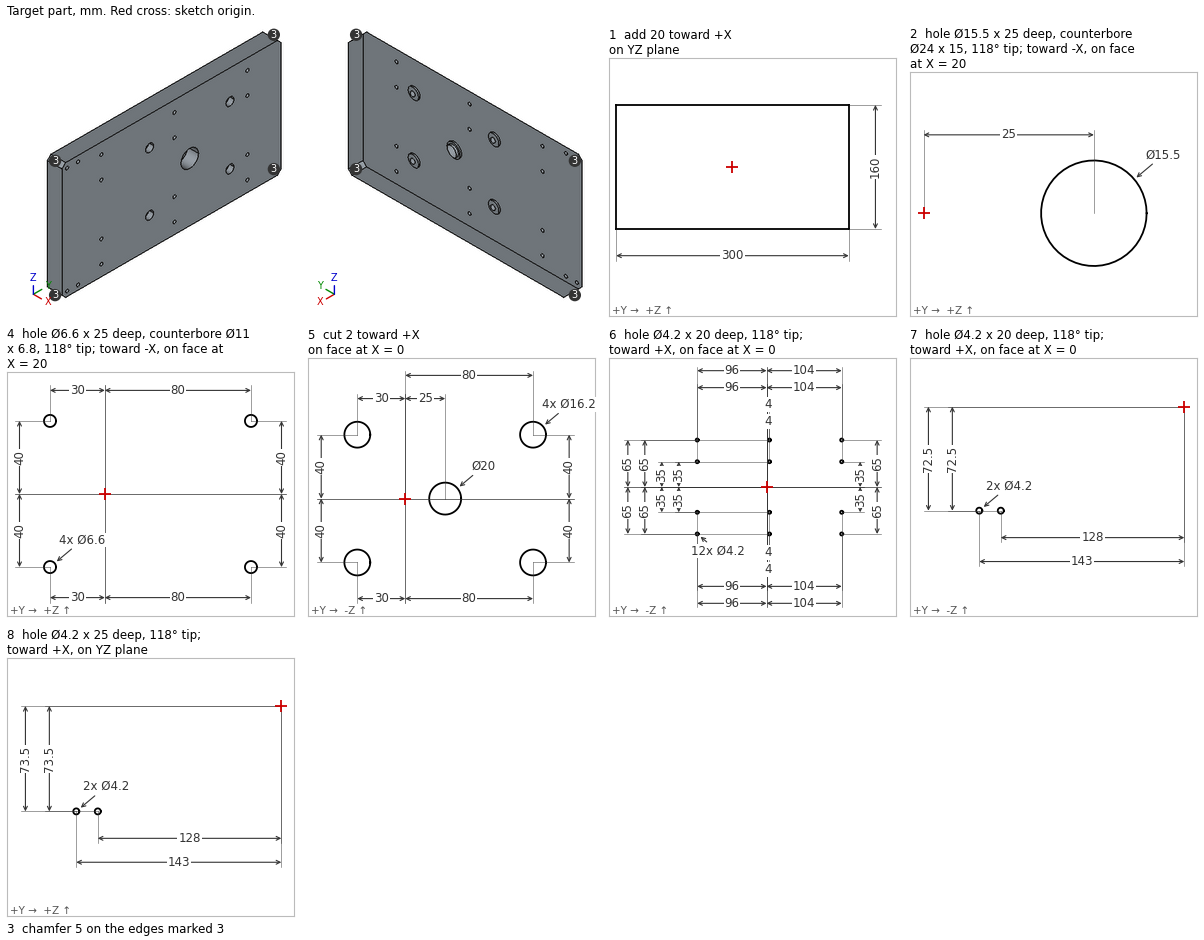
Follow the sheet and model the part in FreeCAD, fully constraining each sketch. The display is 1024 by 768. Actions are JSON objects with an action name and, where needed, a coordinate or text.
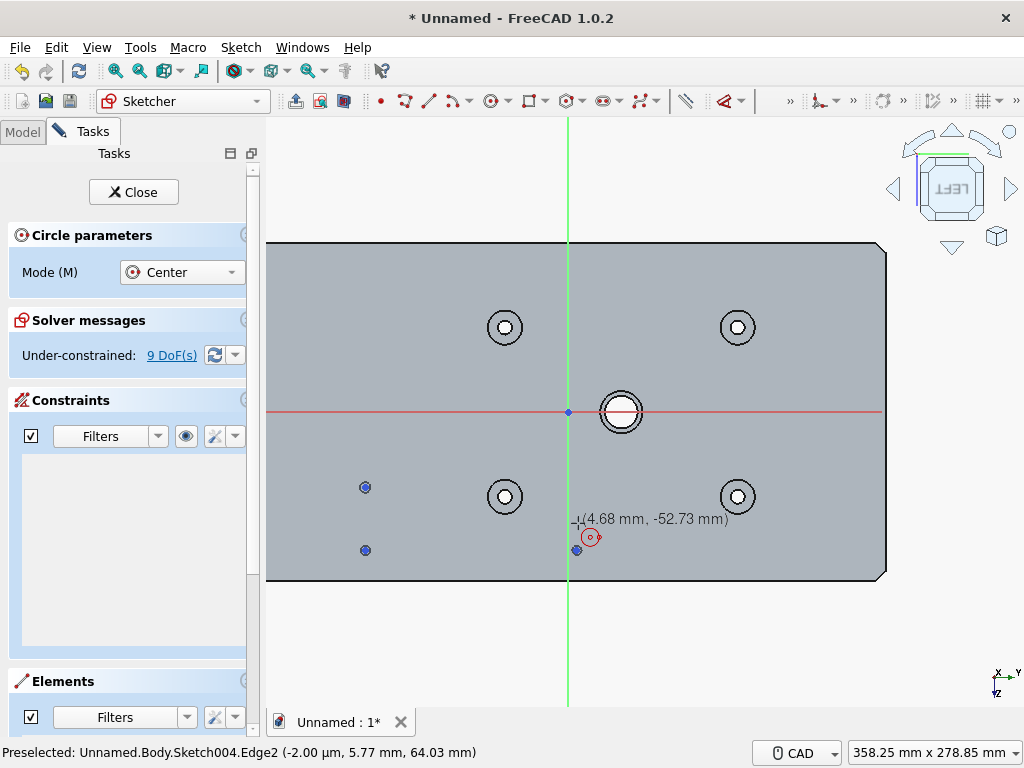
{"action": "scroll", "coordinate": [577, 486], "scroll_direction": "up", "scroll_amount": 4}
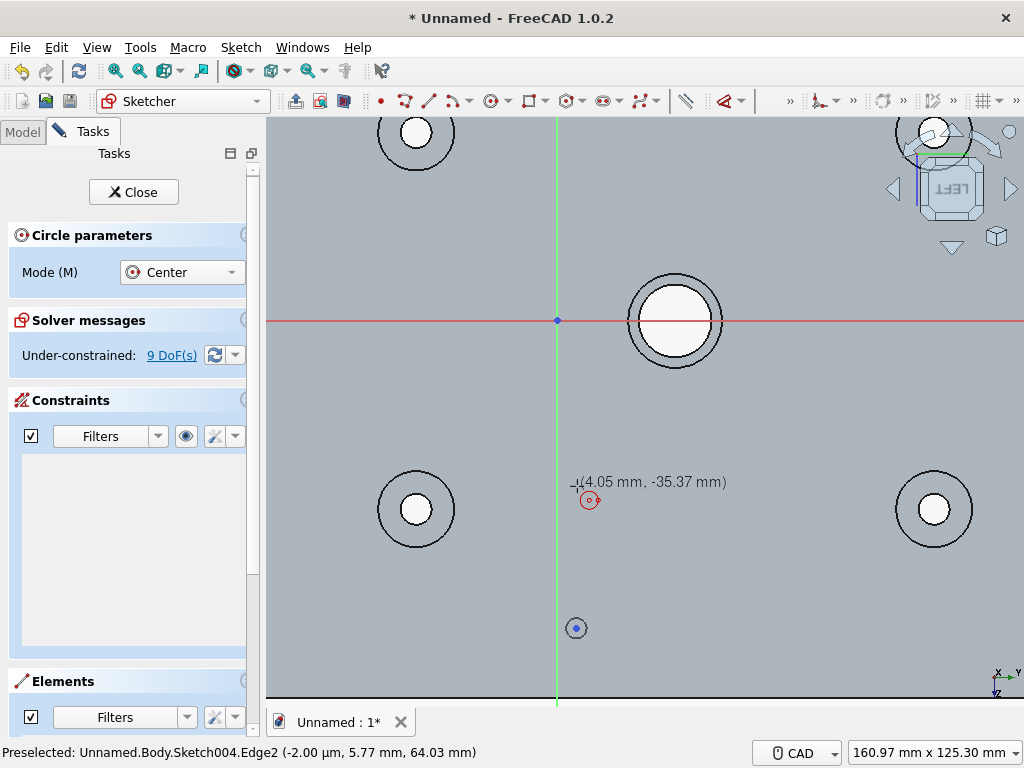
{"action": "left_click", "coordinate": [576, 486]}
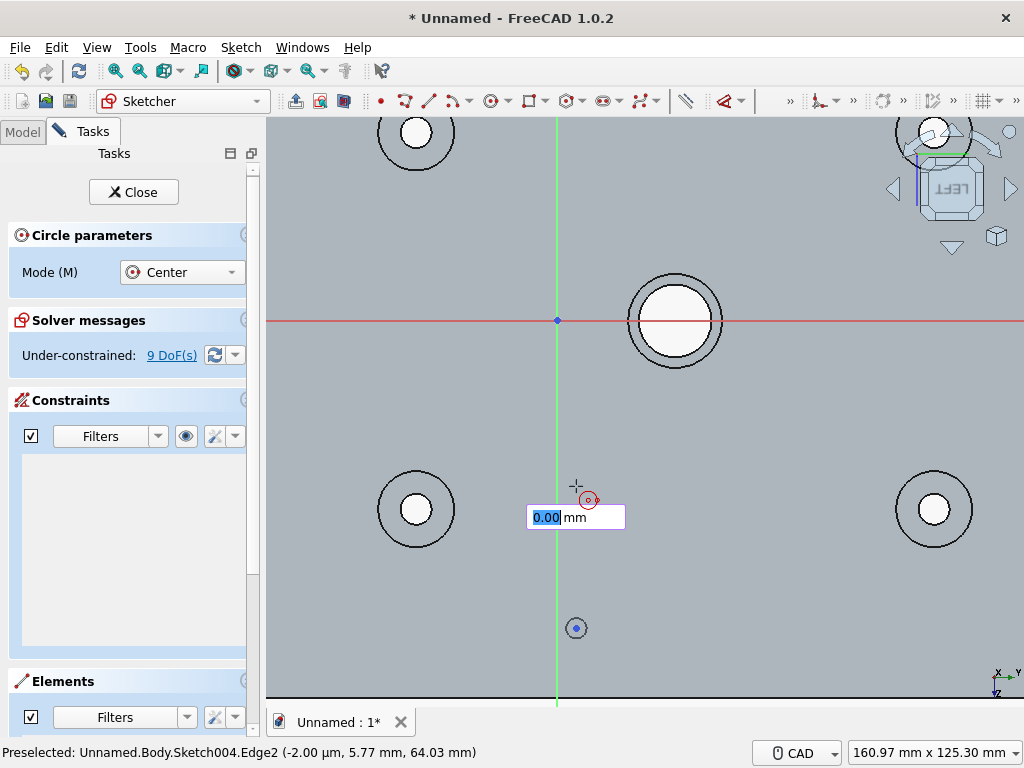
{"action": "scroll", "coordinate": [583, 479], "scroll_direction": "up", "scroll_amount": 3}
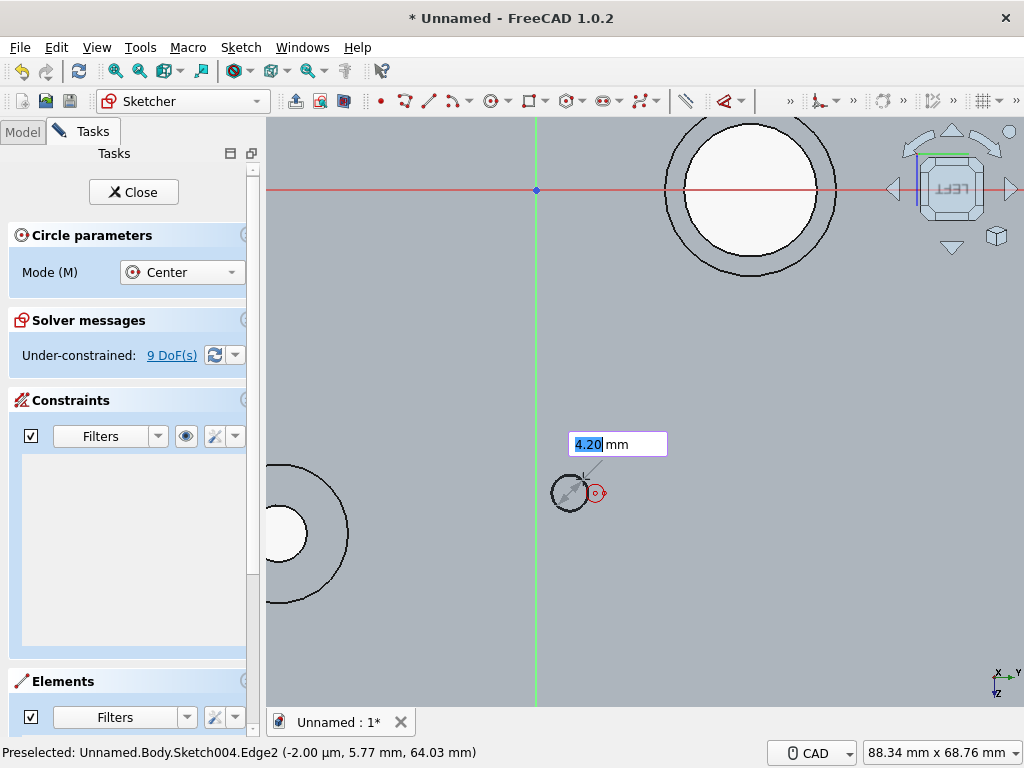
{"action": "left_click", "coordinate": [583, 478]}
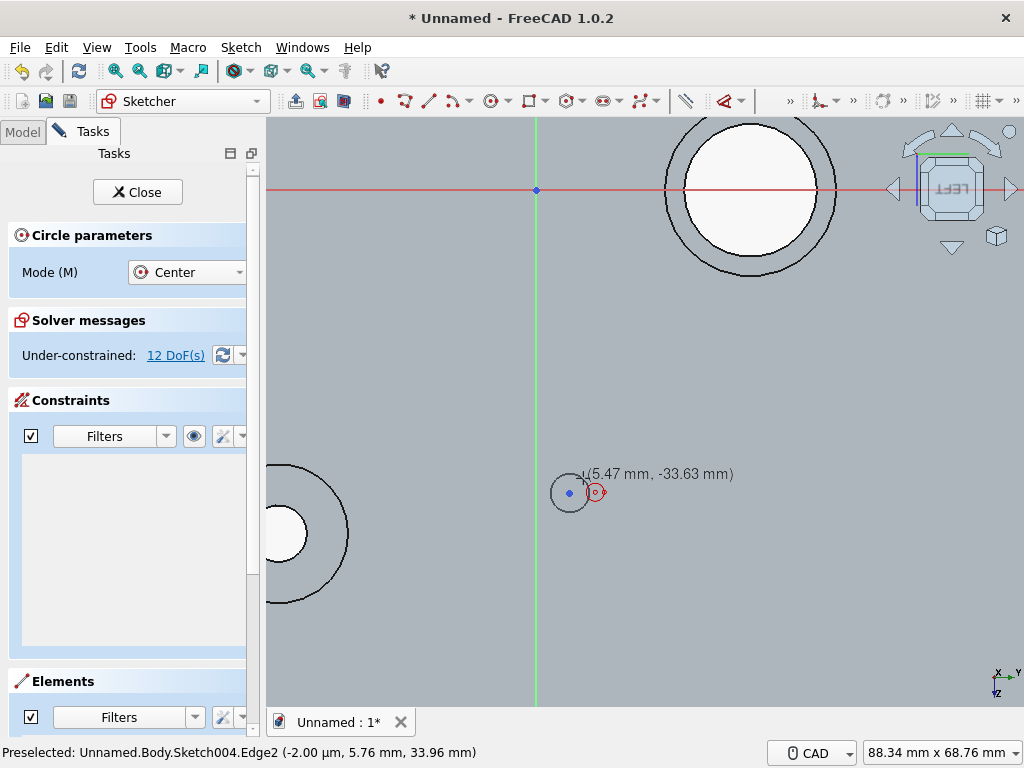
{"action": "scroll", "coordinate": [579, 485], "scroll_direction": "down", "scroll_amount": 7}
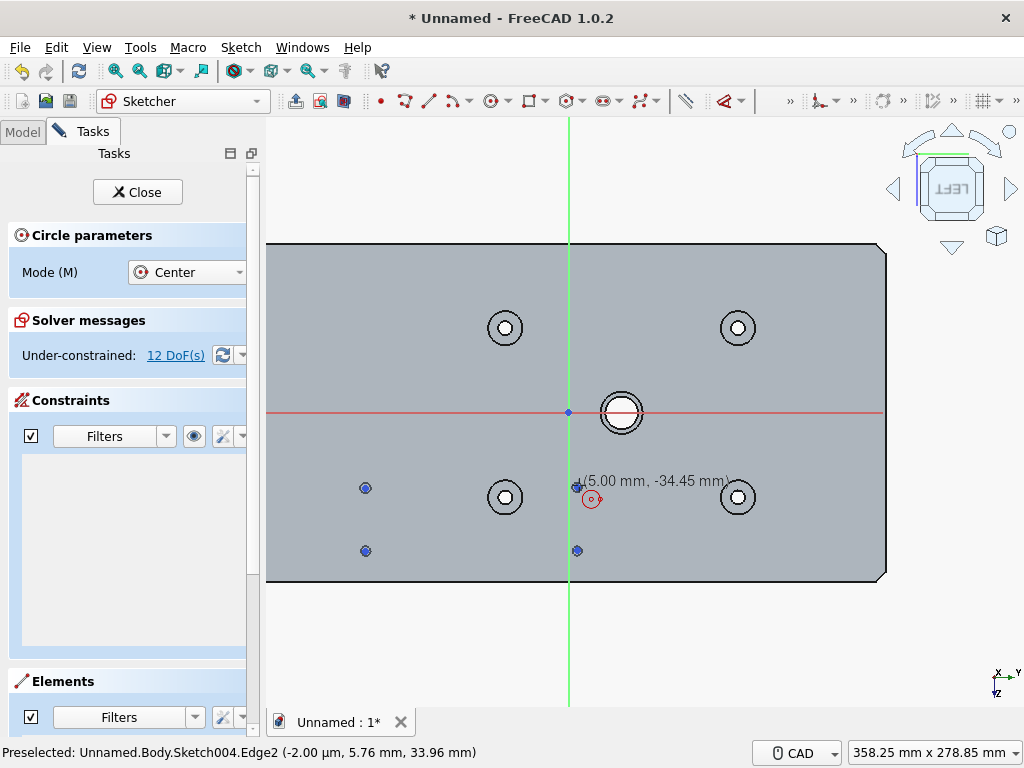
{"action": "scroll", "coordinate": [789, 550], "scroll_direction": "up", "scroll_amount": 9}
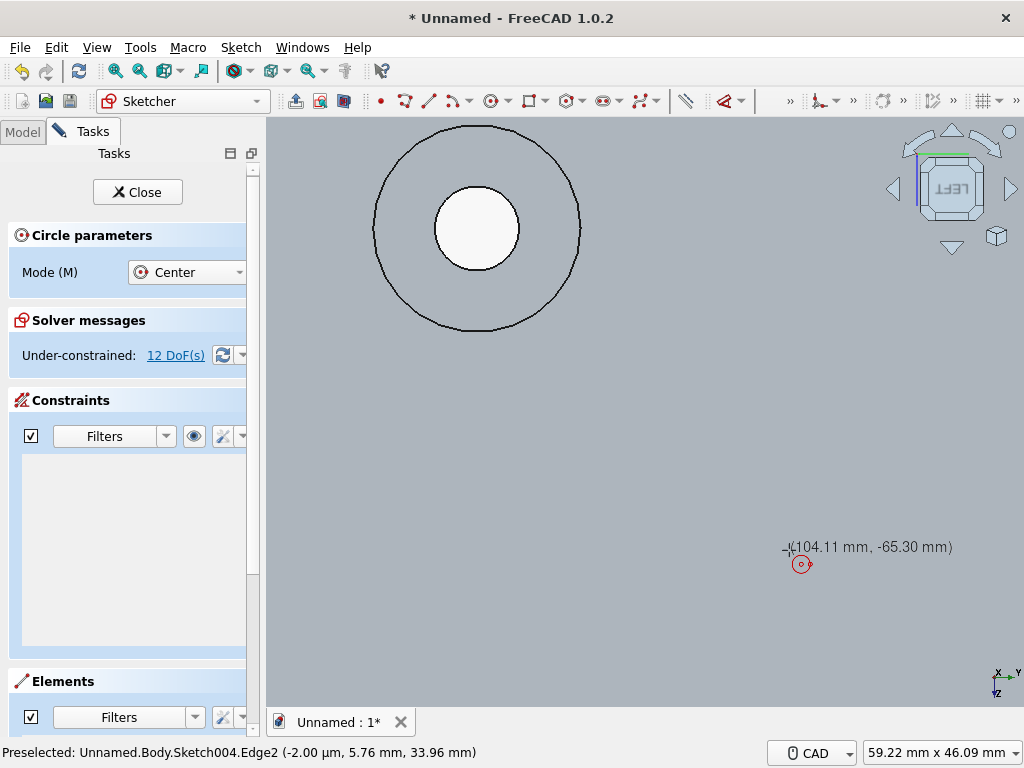
{"action": "scroll", "coordinate": [789, 550], "scroll_direction": "down", "scroll_amount": 9}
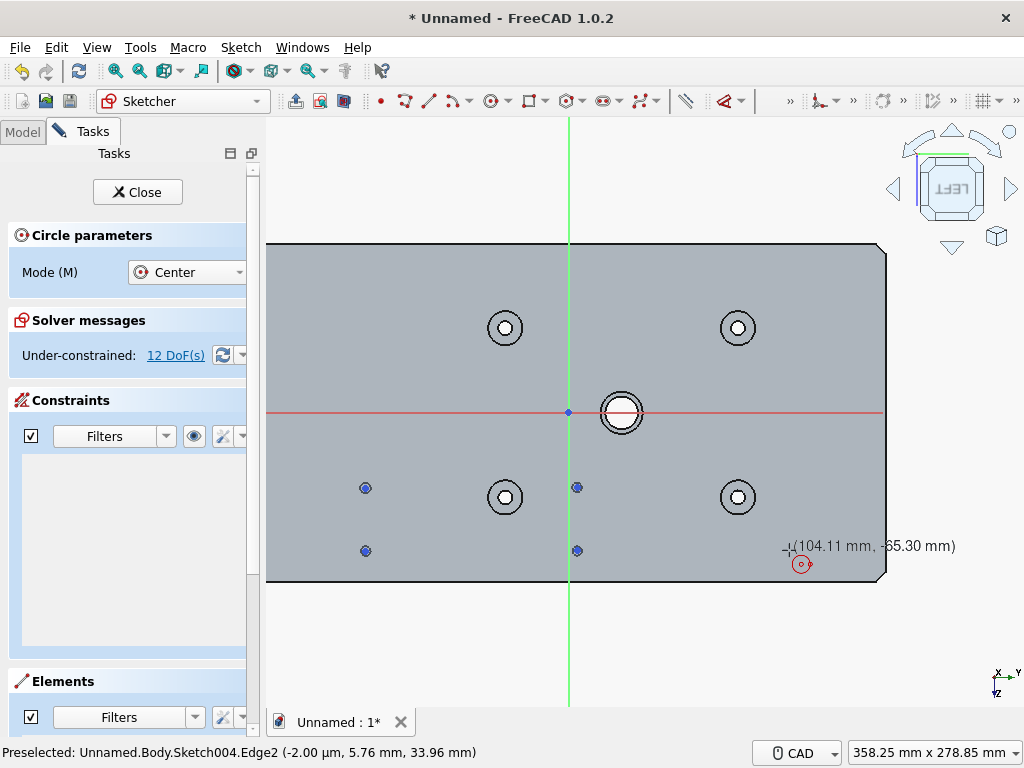
{"action": "left_click", "coordinate": [789, 550]}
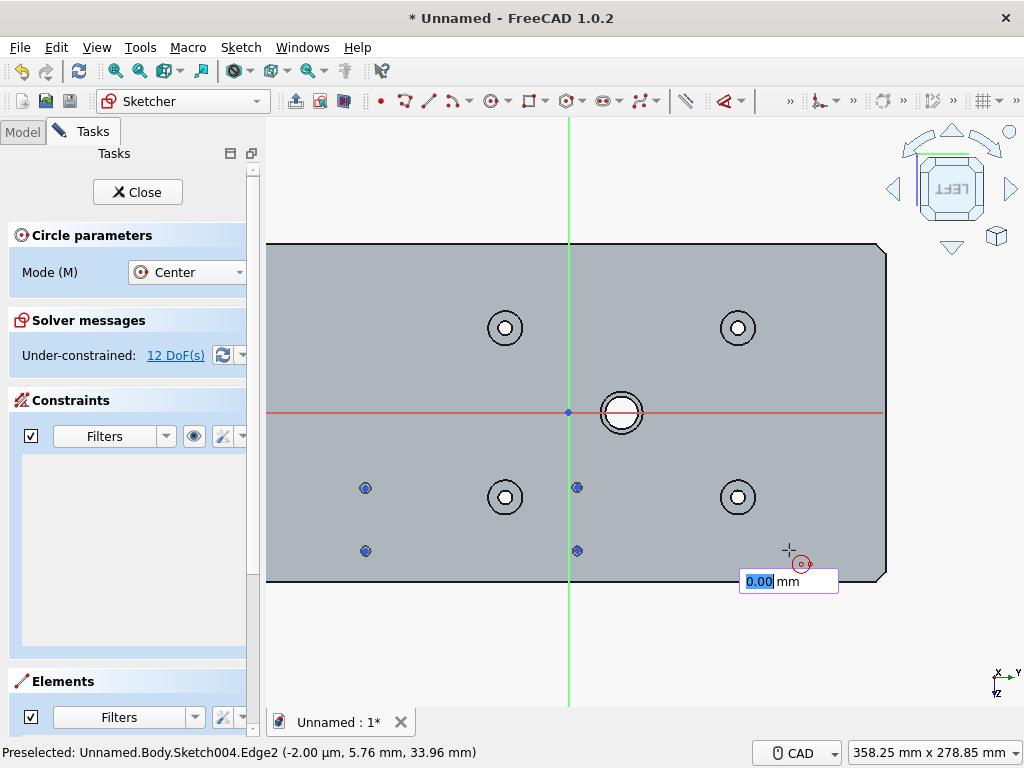
{"action": "scroll", "coordinate": [792, 547], "scroll_direction": "up", "scroll_amount": 7}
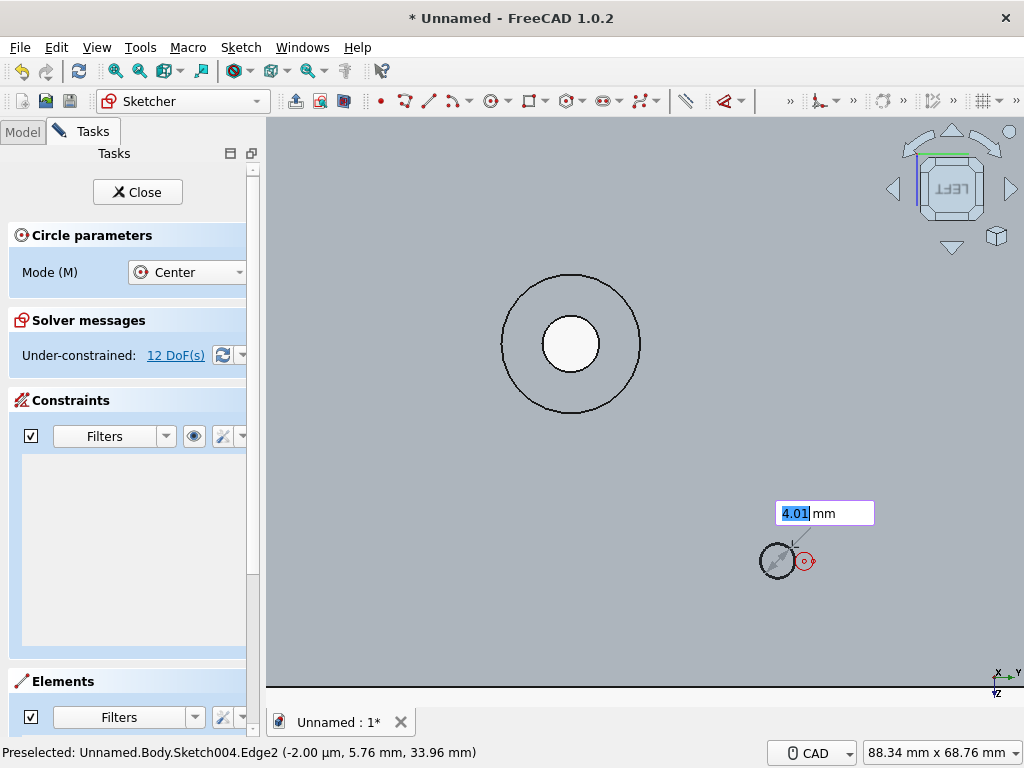
{"action": "left_click", "coordinate": [790, 546]}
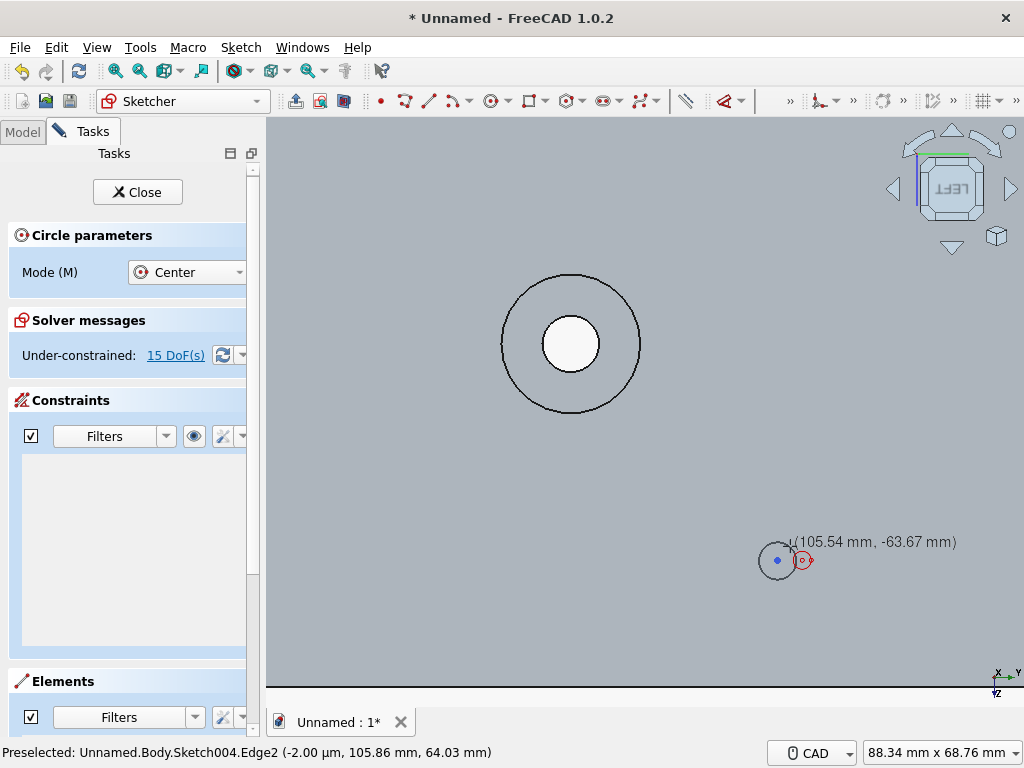
{"action": "scroll", "coordinate": [777, 301], "scroll_direction": "up", "scroll_amount": 2}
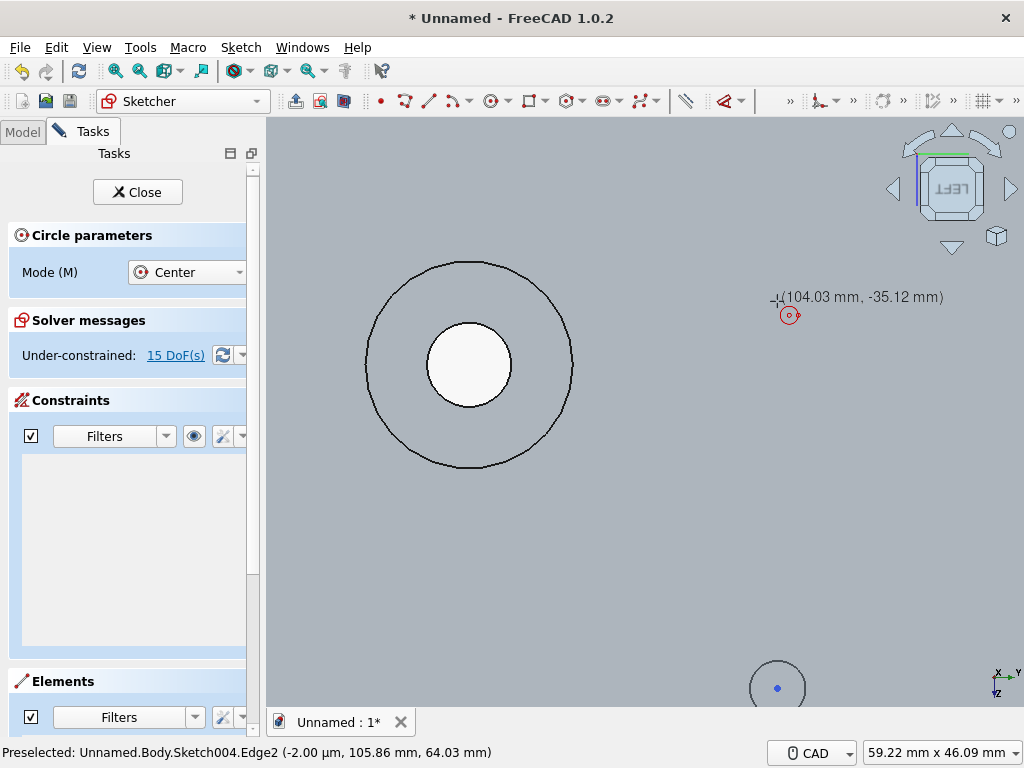
{"action": "scroll", "coordinate": [790, 523], "scroll_direction": "down", "scroll_amount": 9}